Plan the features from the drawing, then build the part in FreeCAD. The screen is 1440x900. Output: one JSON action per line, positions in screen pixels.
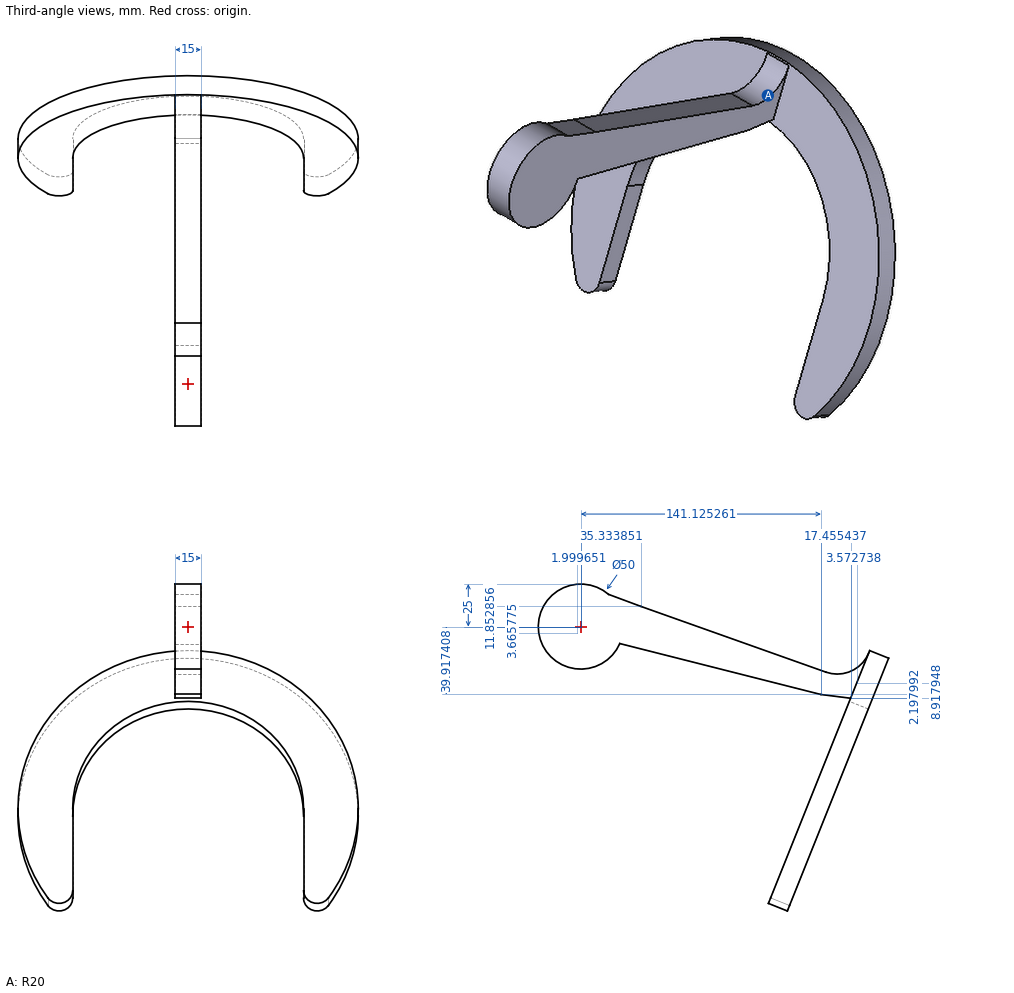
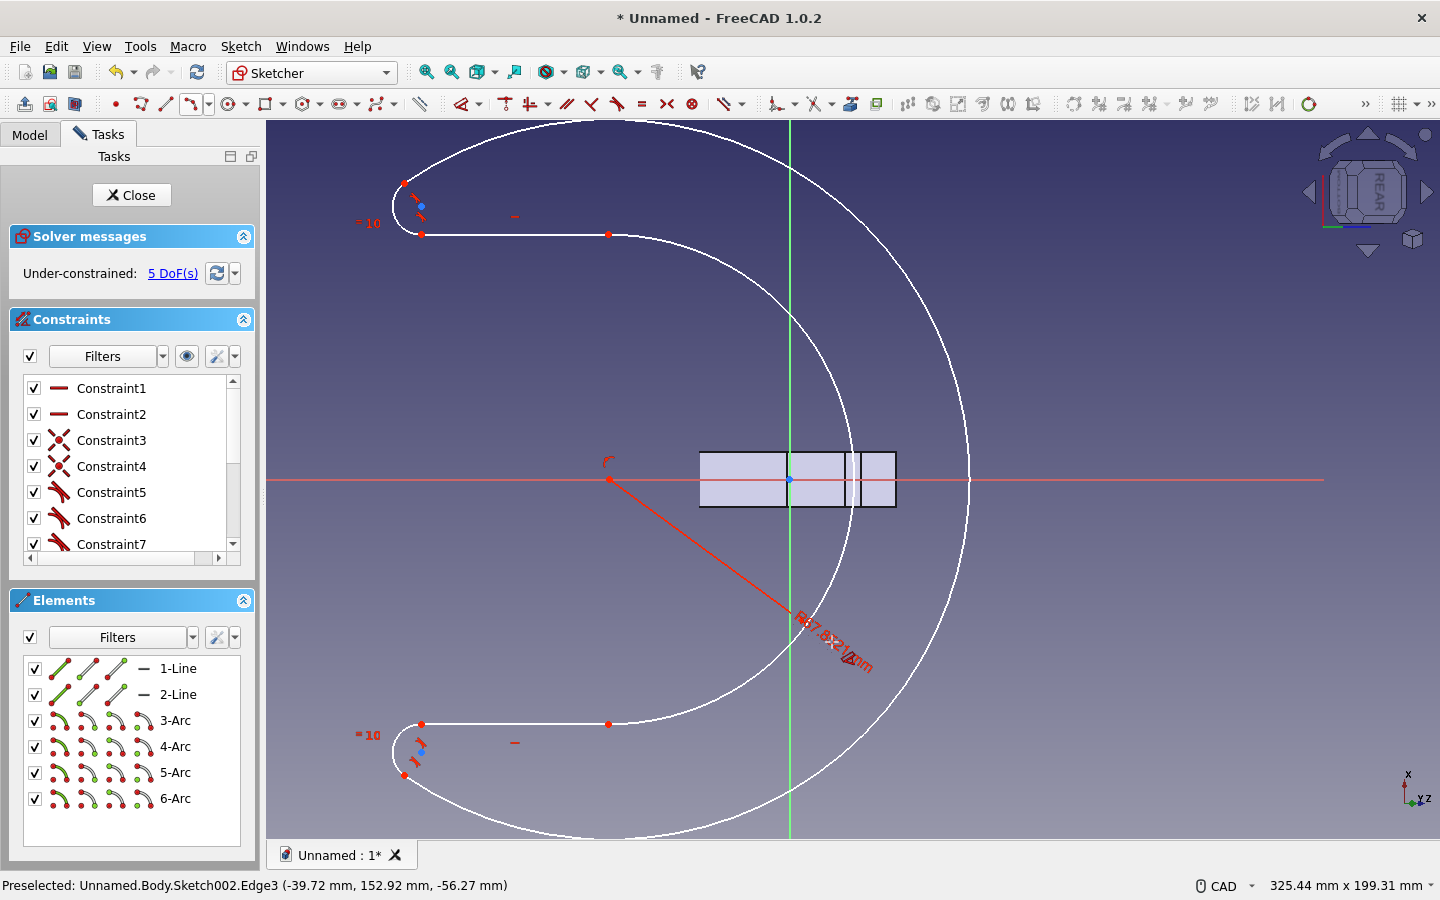
{"action": "scroll", "coordinate": [402, 732], "scroll_direction": "up", "scroll_amount": 2}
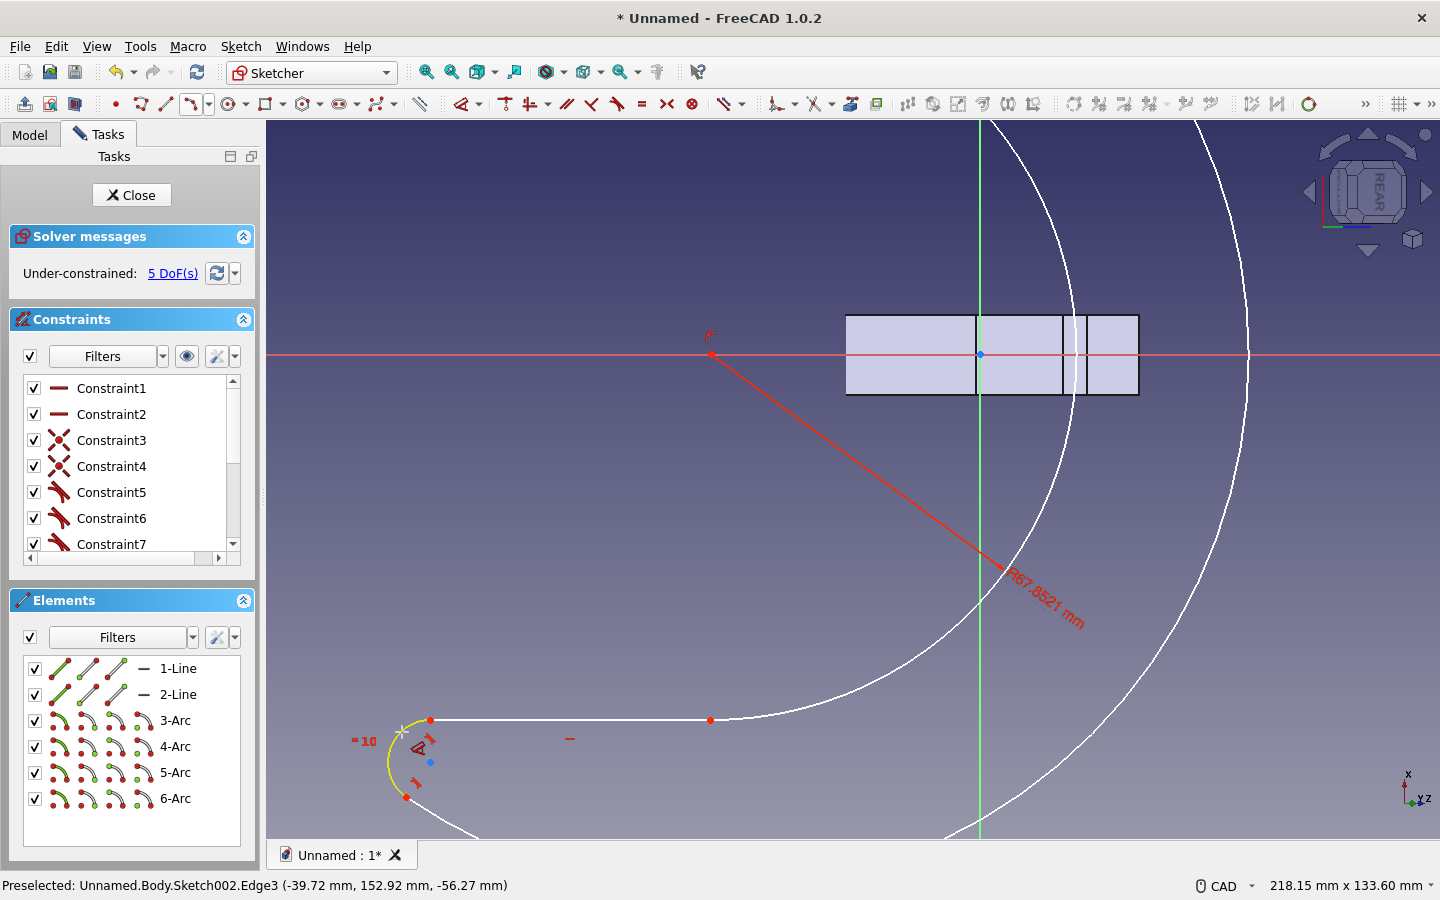
{"action": "left_click", "coordinate": [401, 732]}
{"action": "left_click", "coordinate": [379, 709]}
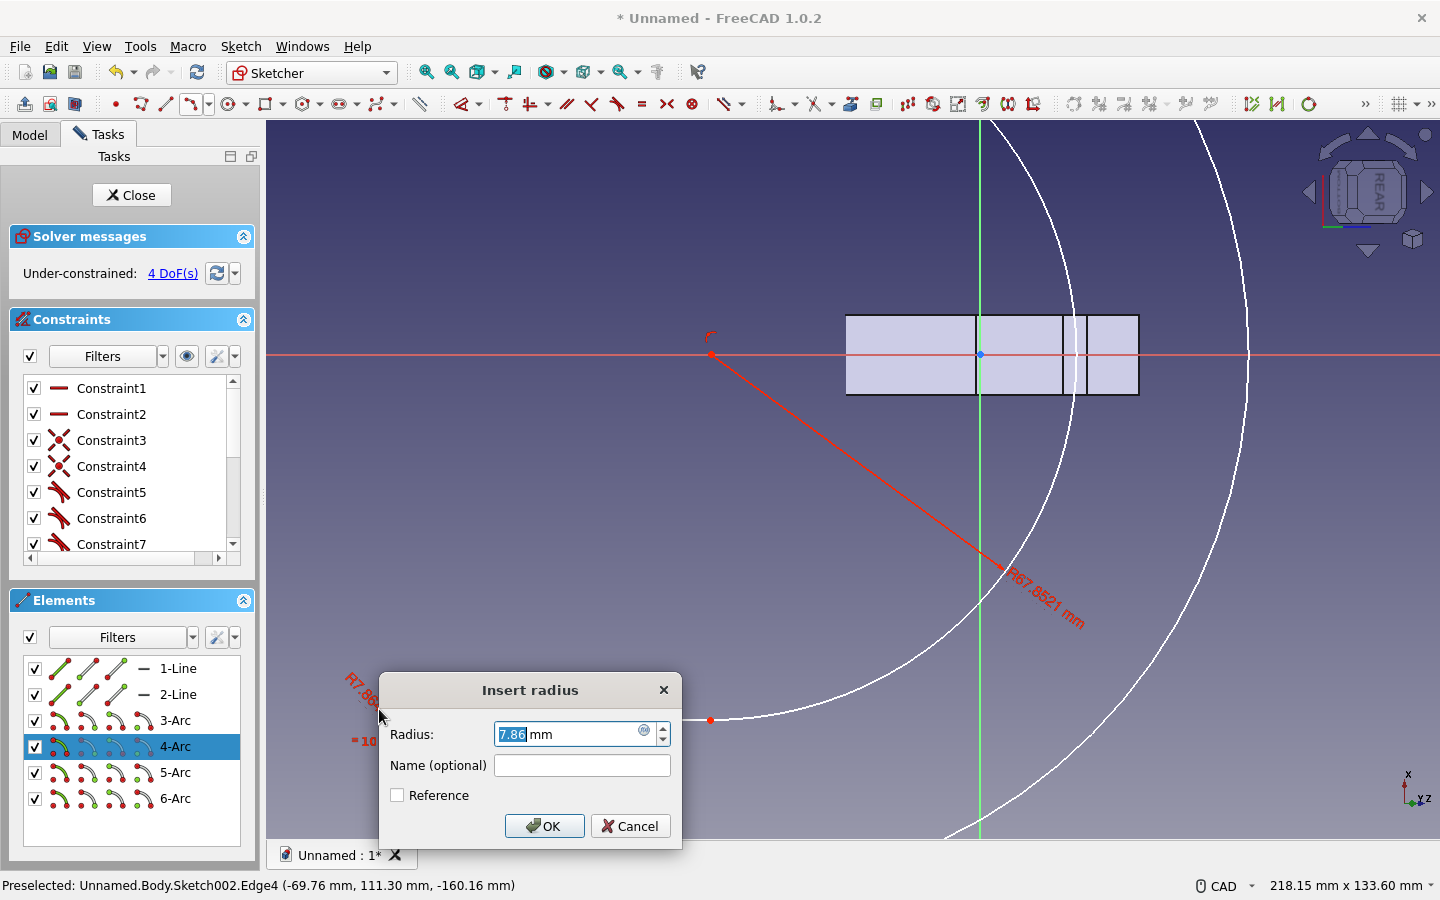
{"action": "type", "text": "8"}
{"action": "key", "text": "Return"}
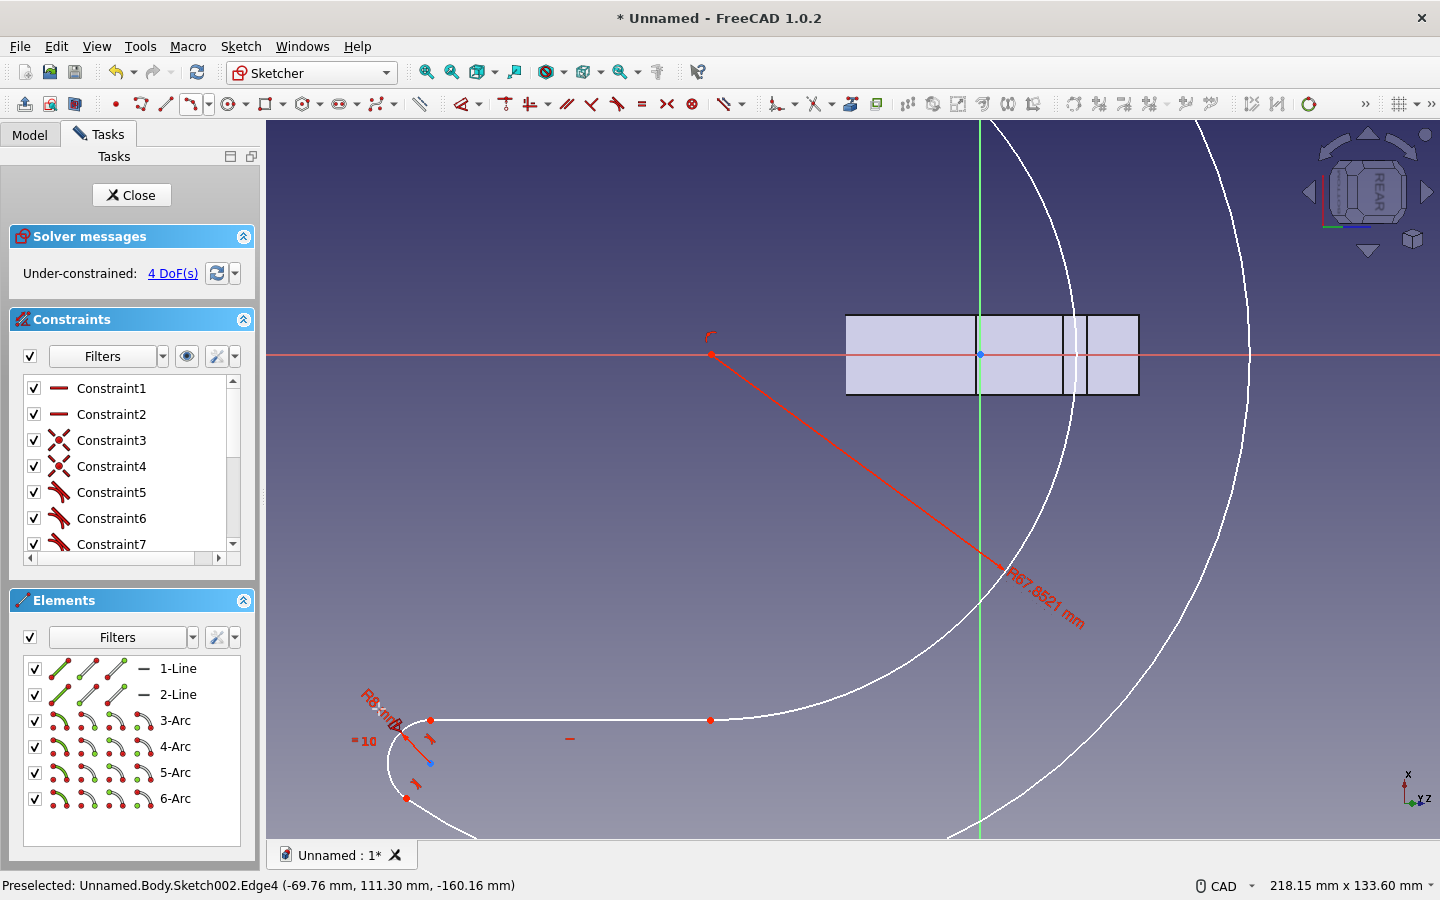
{"action": "left_click", "coordinate": [1059, 766]}
{"action": "left_click", "coordinate": [1080, 790]}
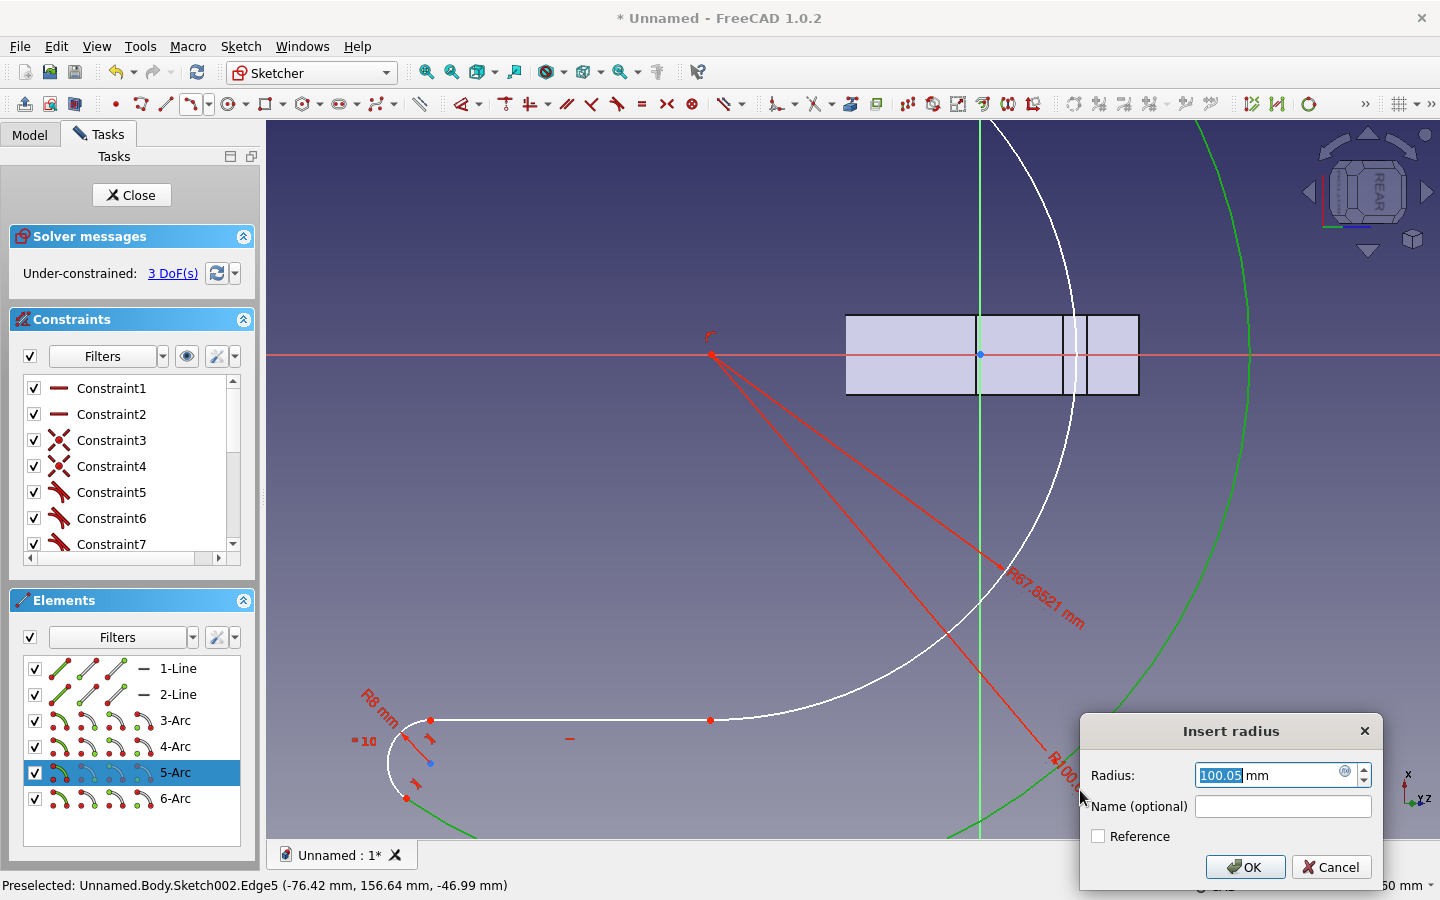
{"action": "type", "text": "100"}
{"action": "key", "text": "Return"}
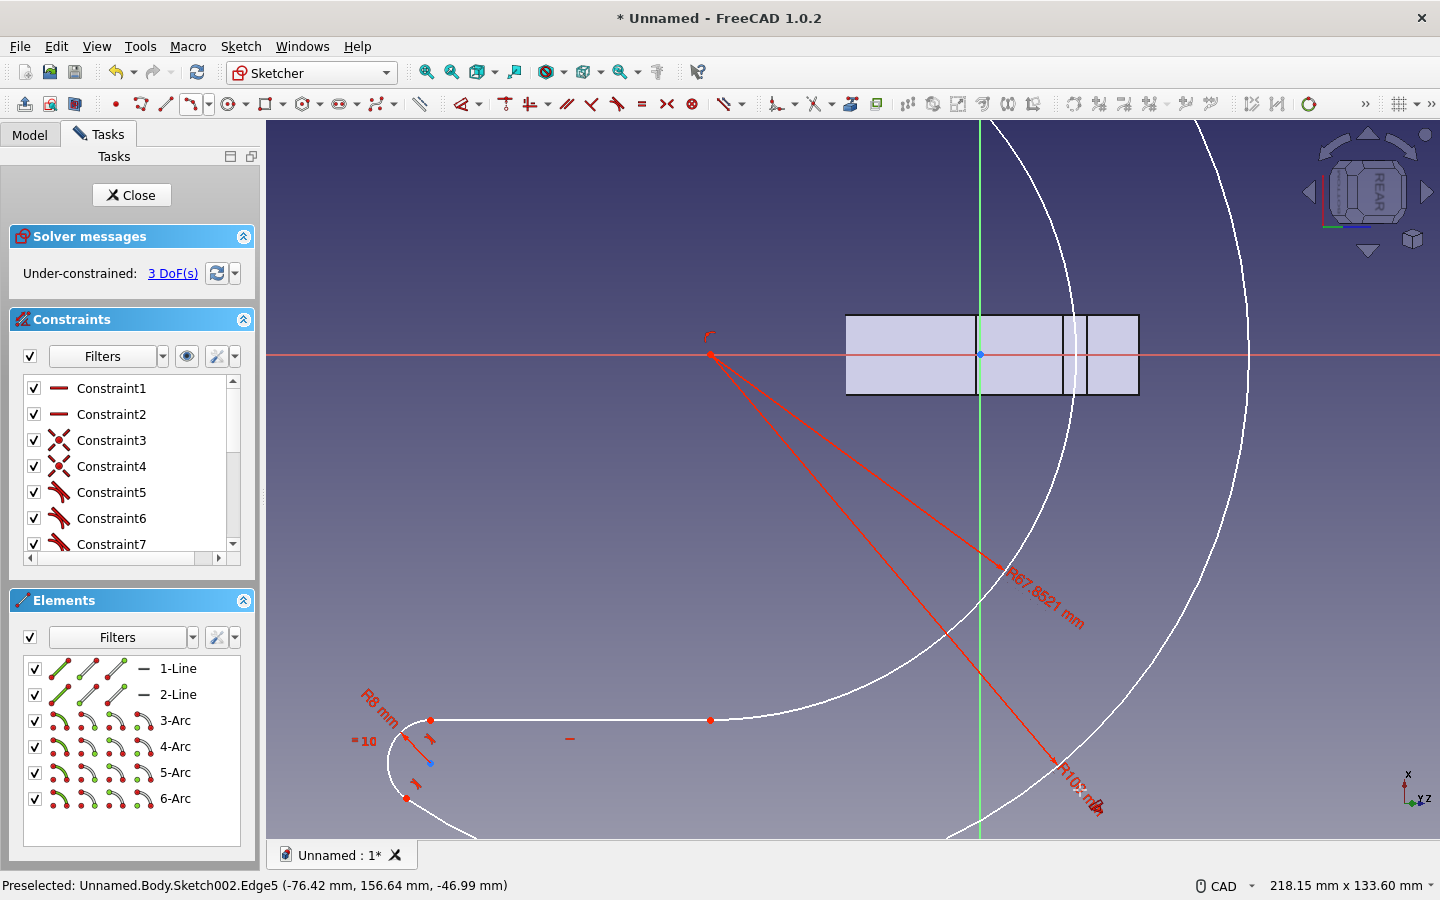
{"action": "scroll", "coordinate": [742, 631], "scroll_direction": "down", "scroll_amount": 3}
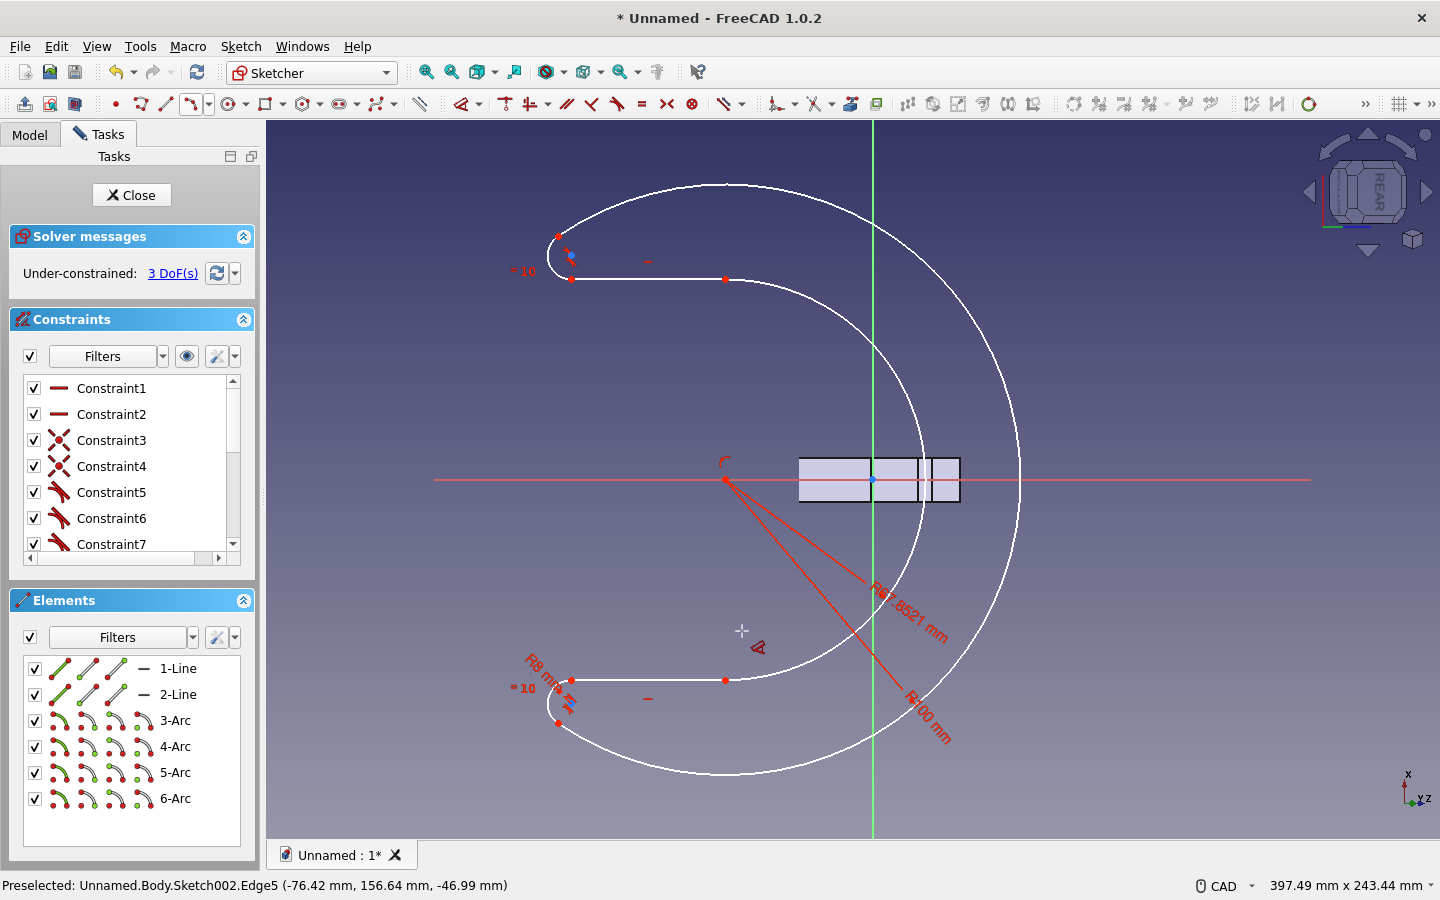
{"action": "left_click", "coordinate": [617, 279]}
{"action": "left_click", "coordinate": [648, 245]}